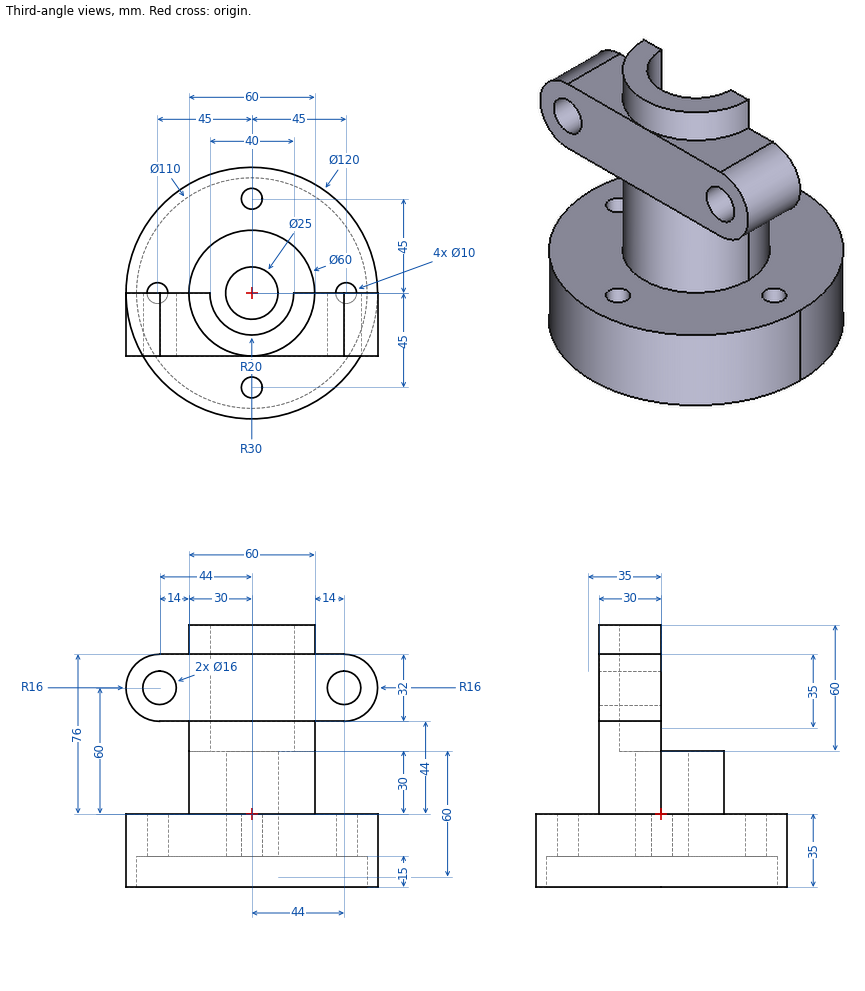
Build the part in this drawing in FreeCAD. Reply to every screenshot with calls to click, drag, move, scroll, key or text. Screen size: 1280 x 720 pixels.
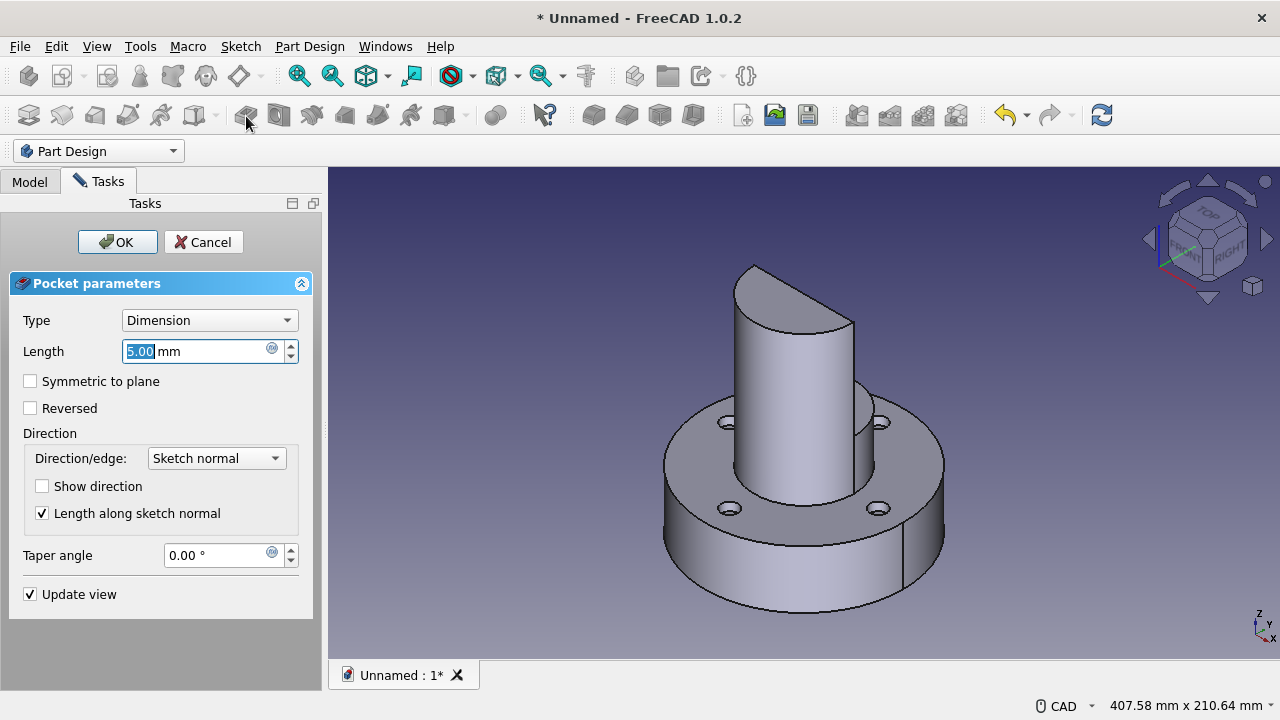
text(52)
key(Tab)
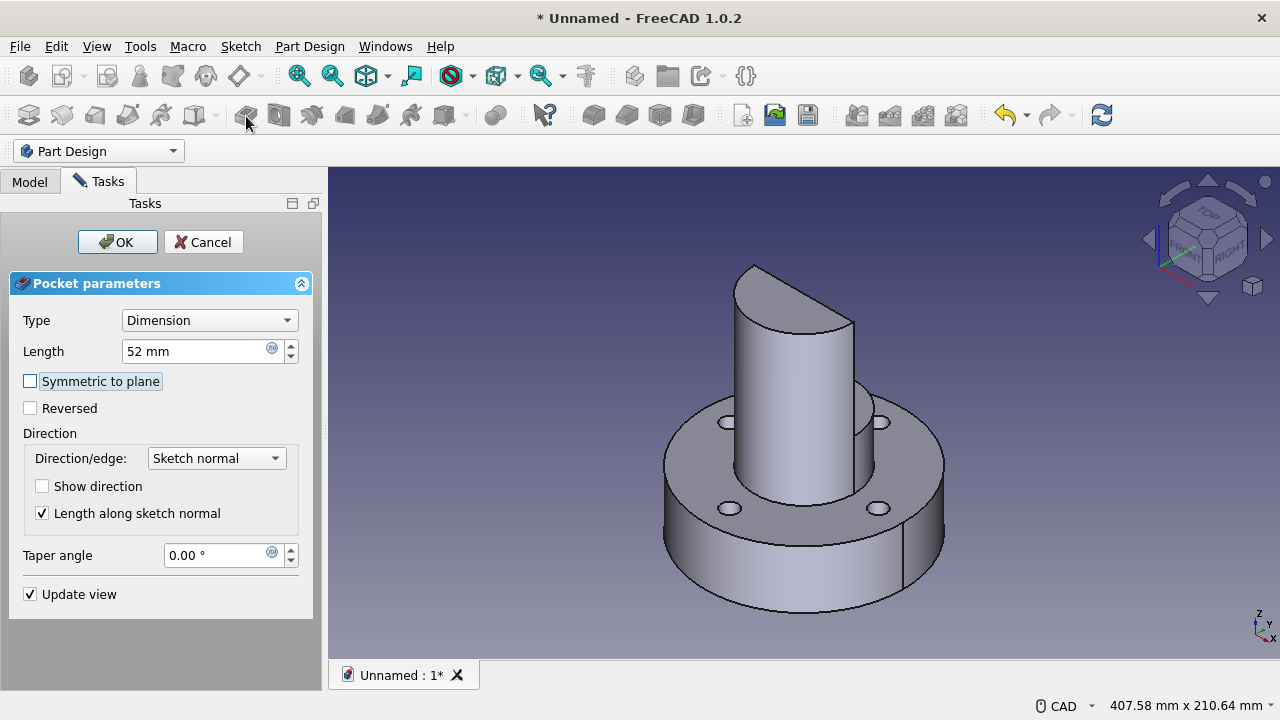
click(118, 242)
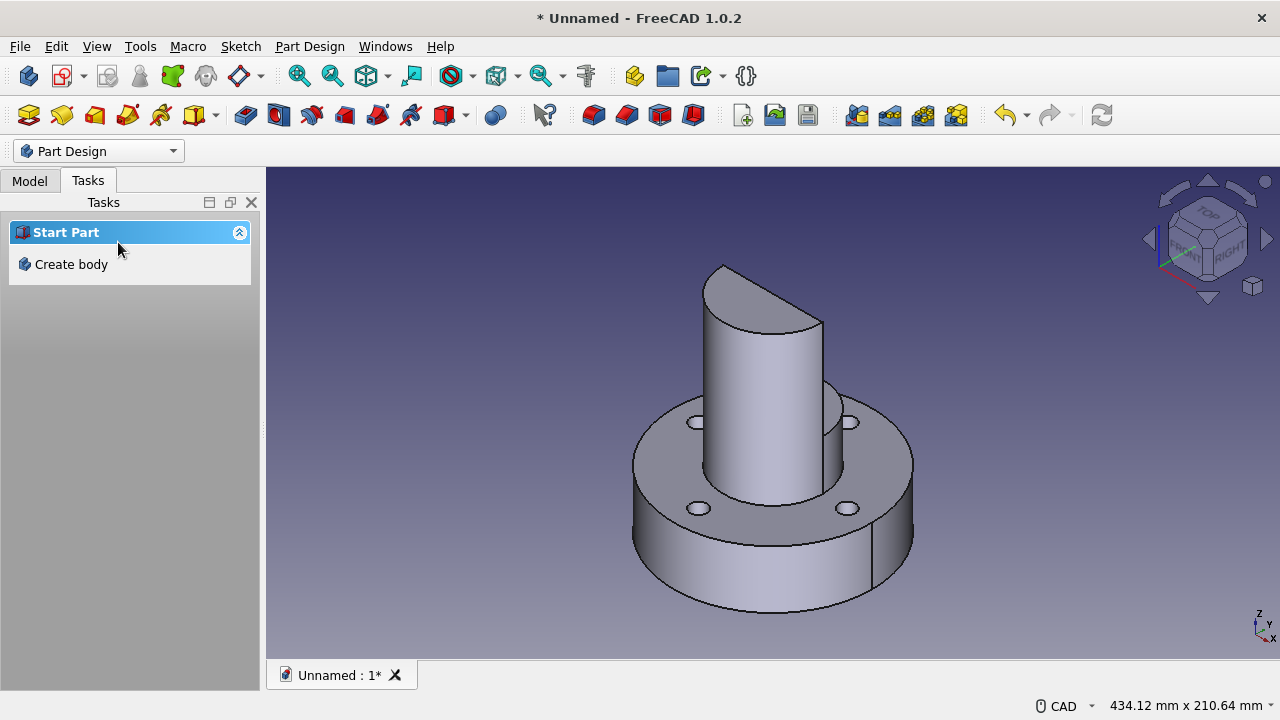
click(748, 307)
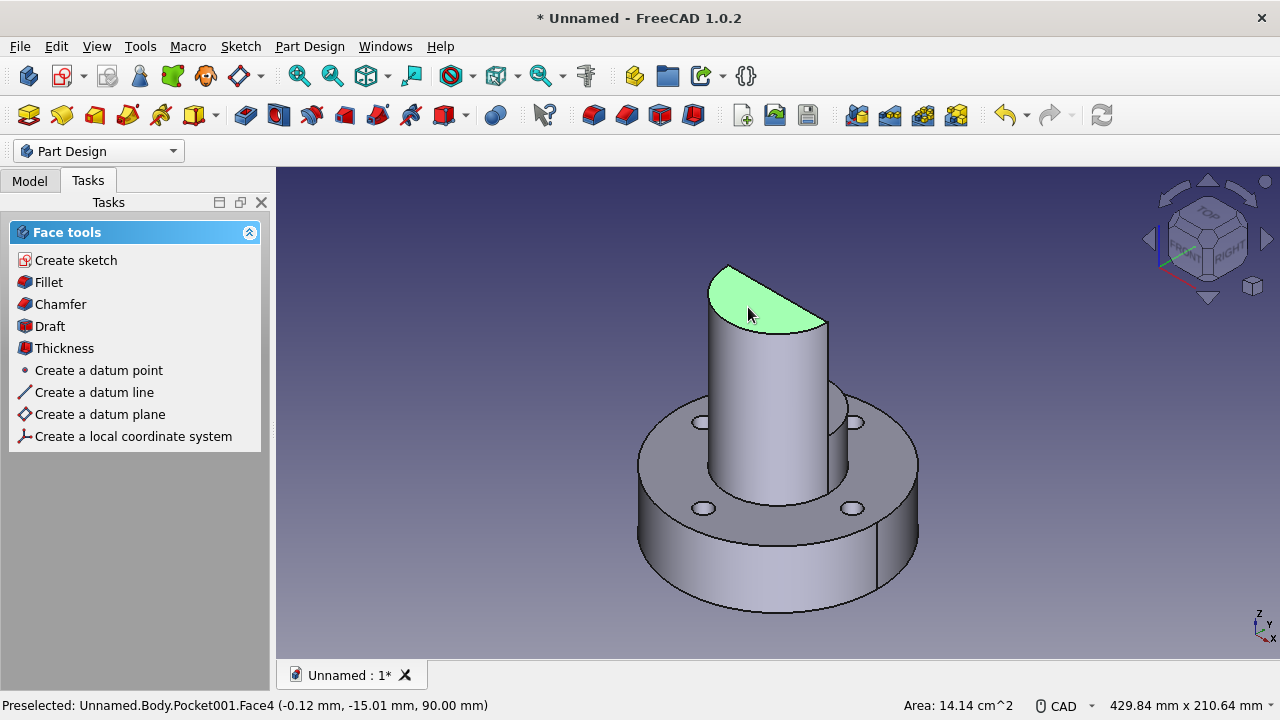
click(62, 76)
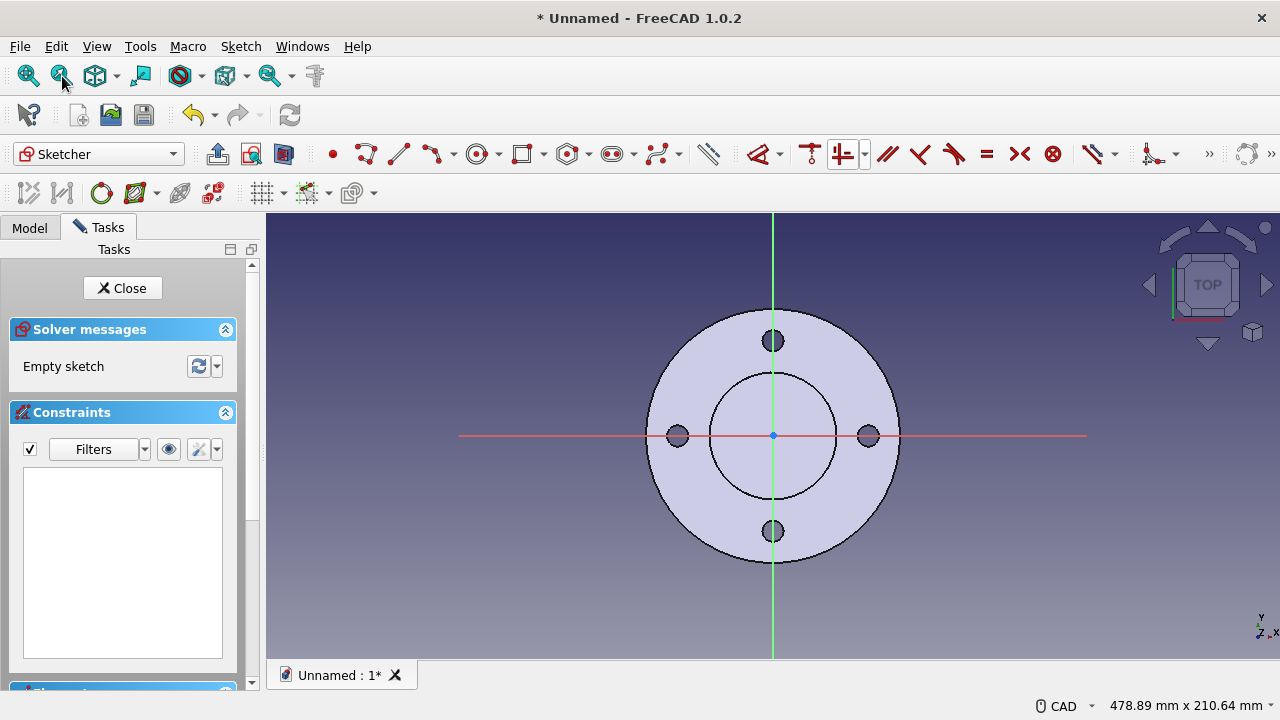
scroll(787, 461, up, 9)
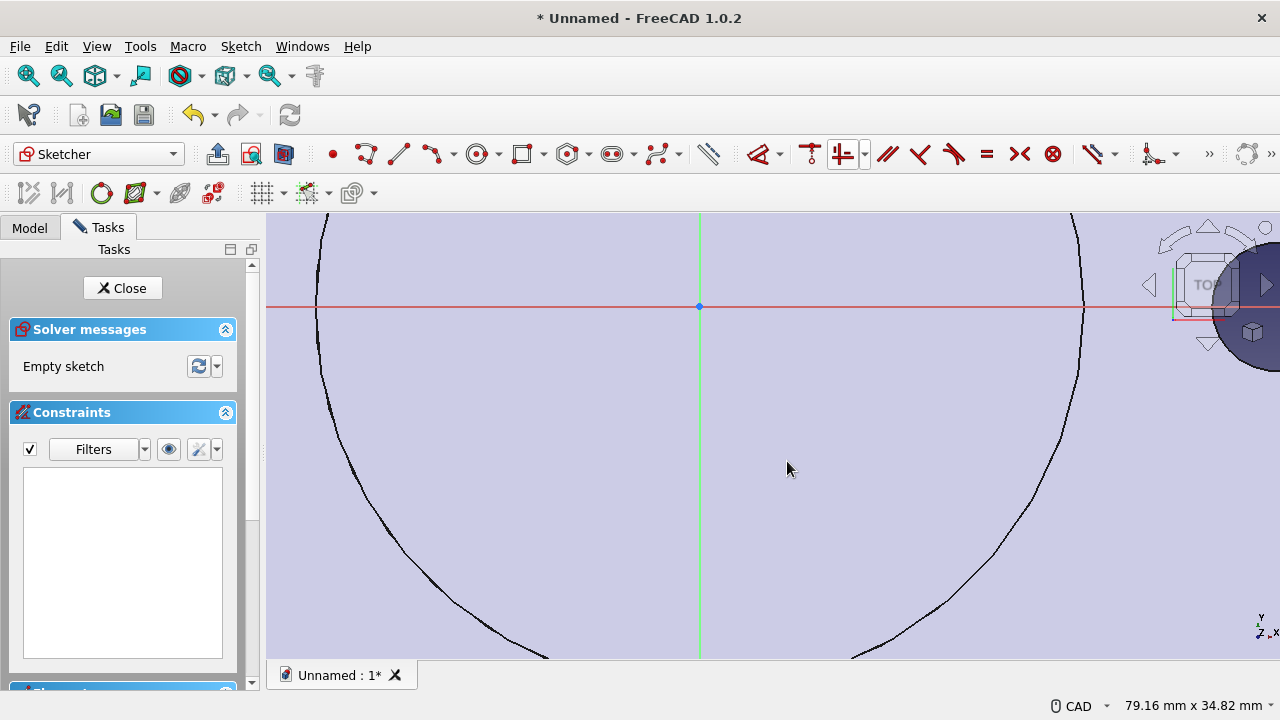
click(399, 154)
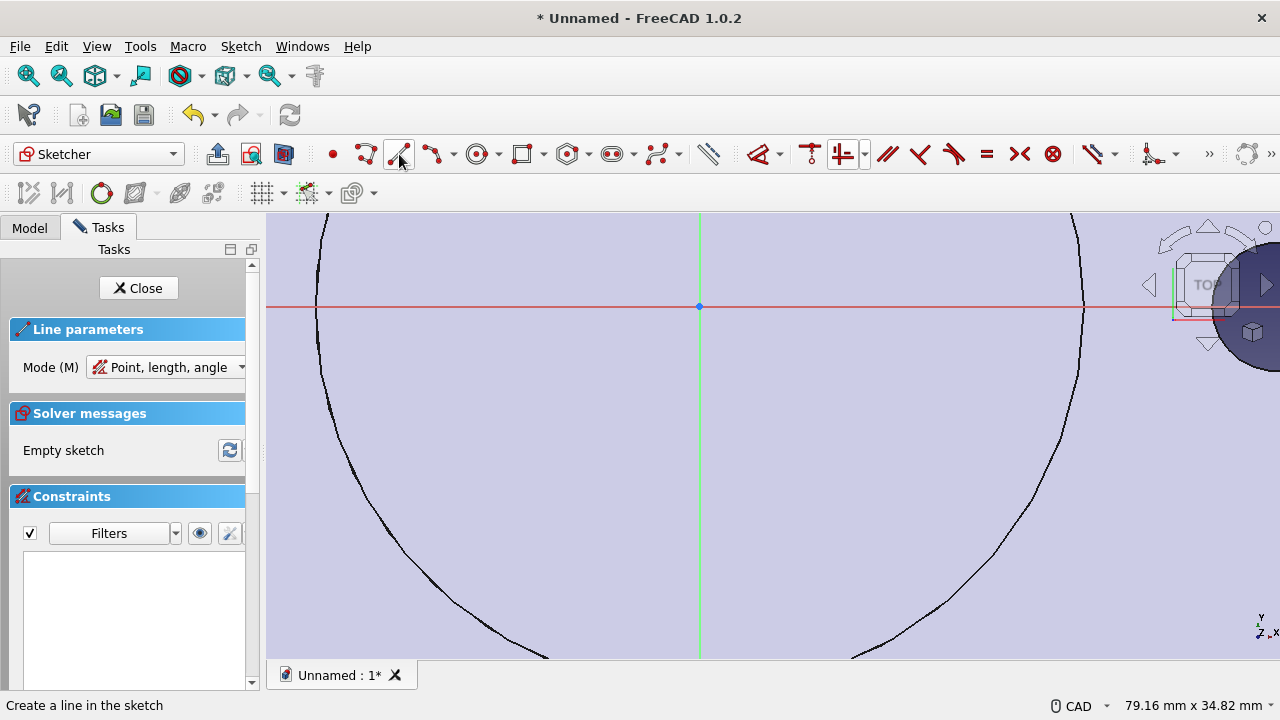
click(956, 307)
click(444, 316)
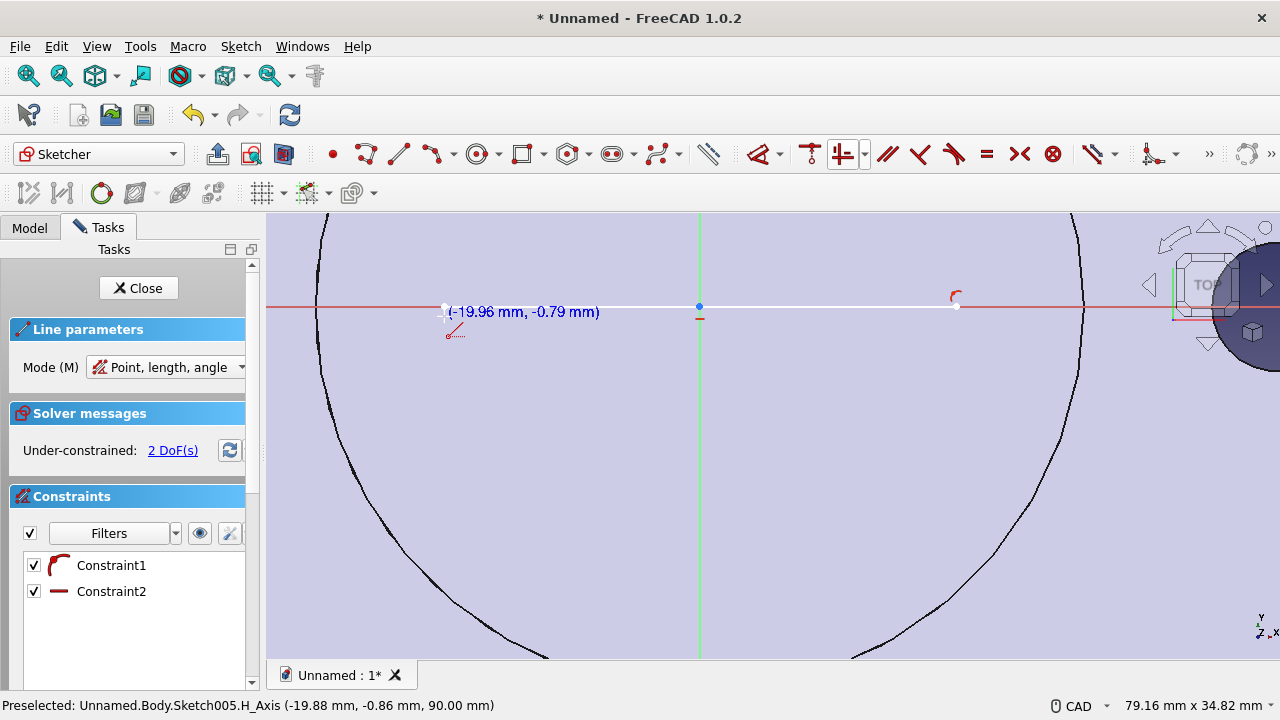
click(432, 154)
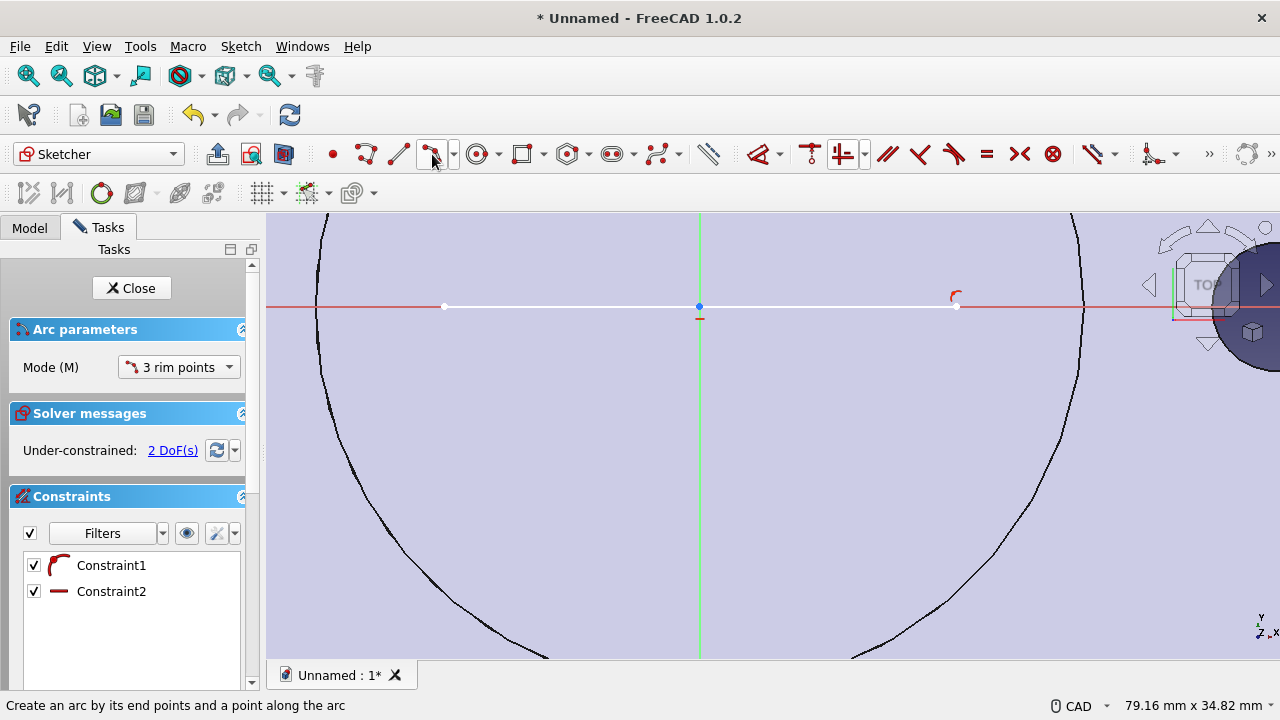
click(444, 316)
click(956, 307)
click(621, 551)
key(Escape)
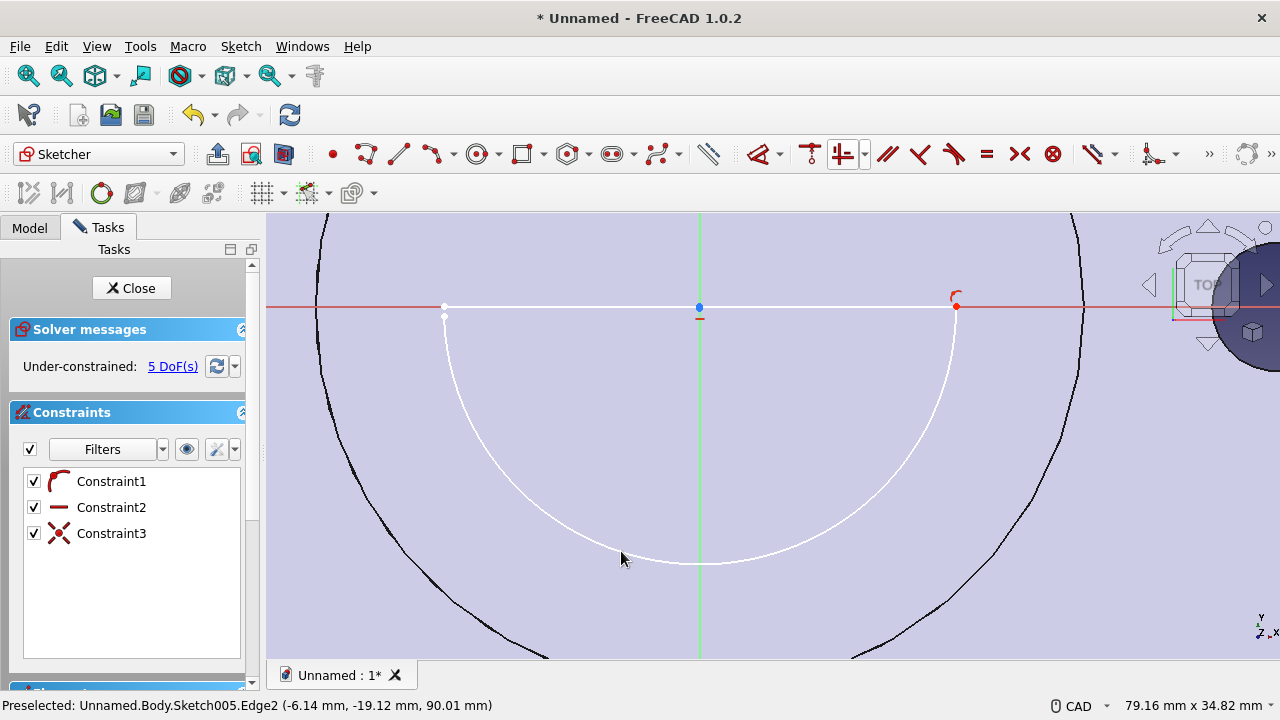
drag(690, 297, 710, 318)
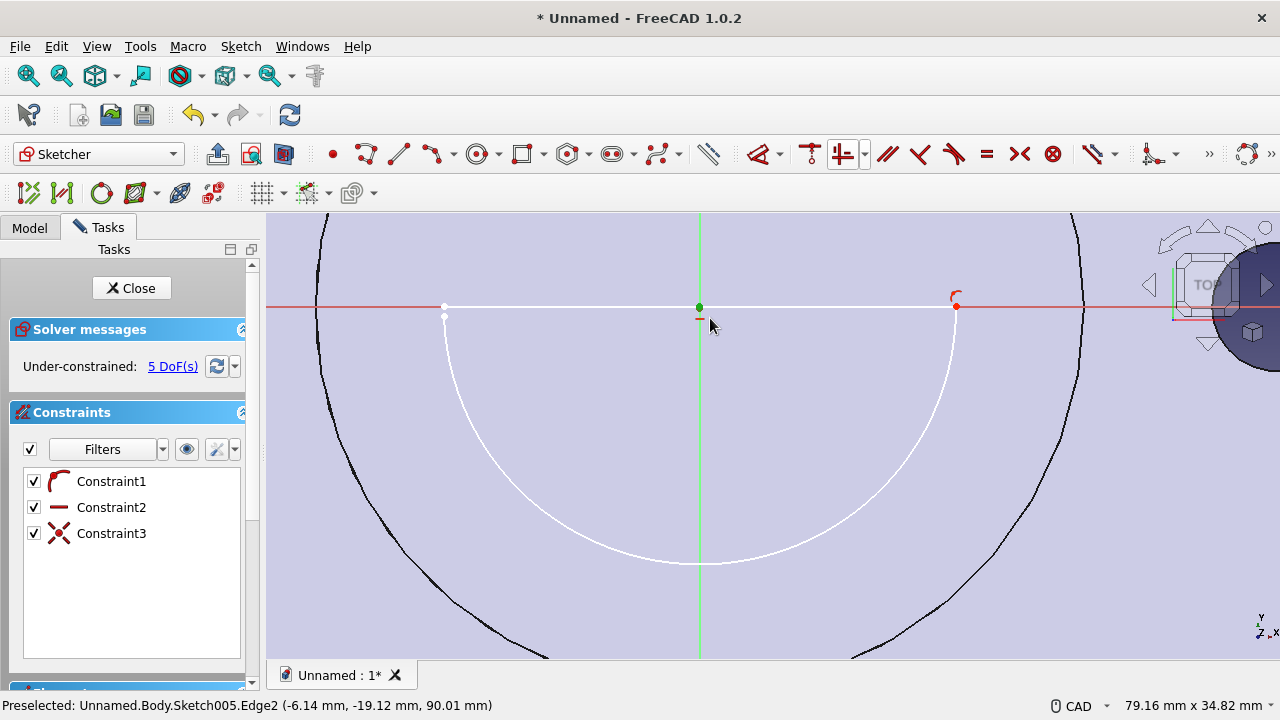
click(810, 154)